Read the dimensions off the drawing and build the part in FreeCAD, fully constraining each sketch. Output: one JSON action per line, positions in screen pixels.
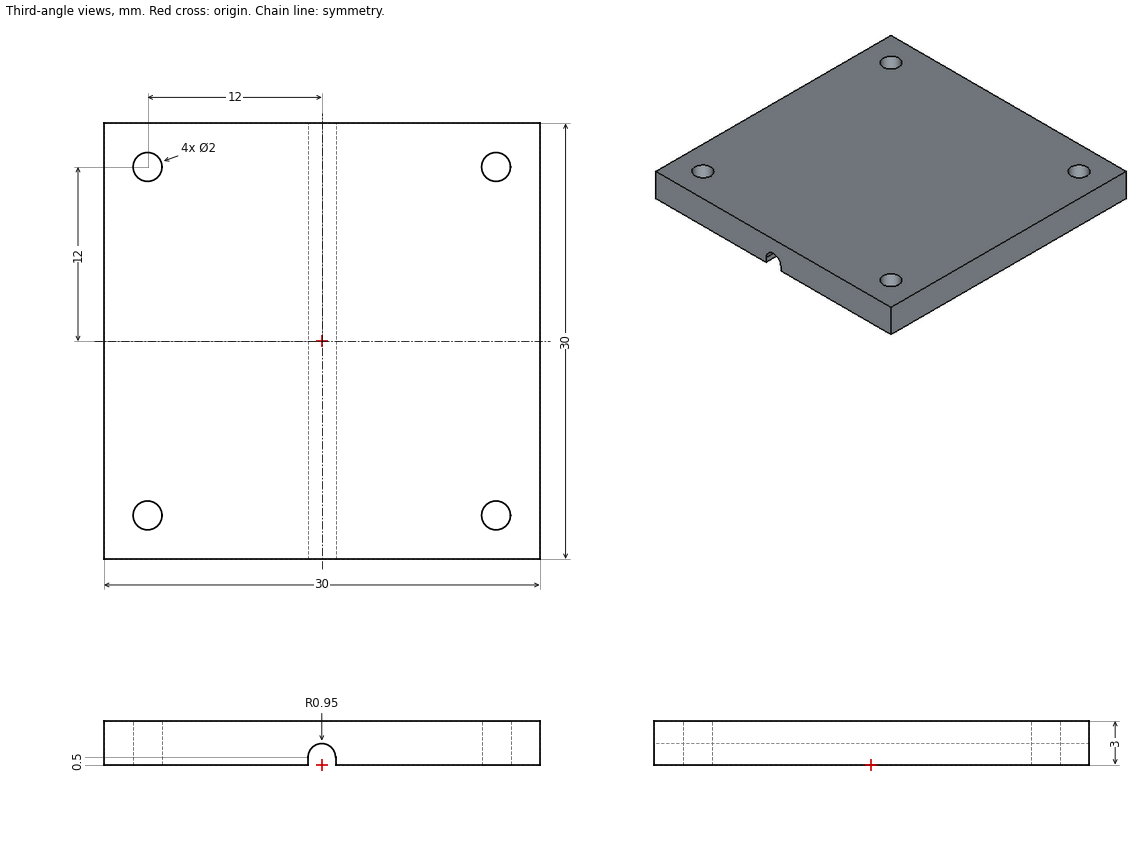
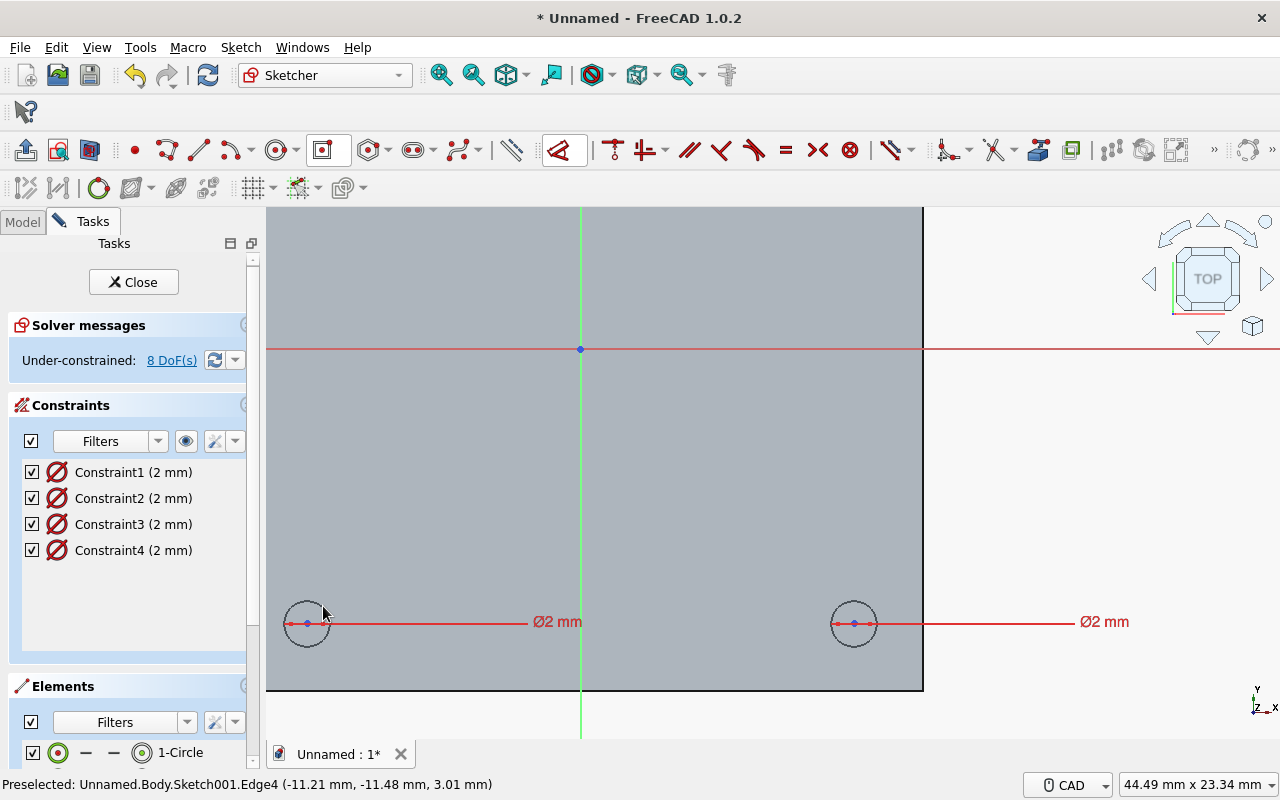
{"action": "scroll", "coordinate": [855, 624], "scroll_direction": "down", "scroll_amount": 3}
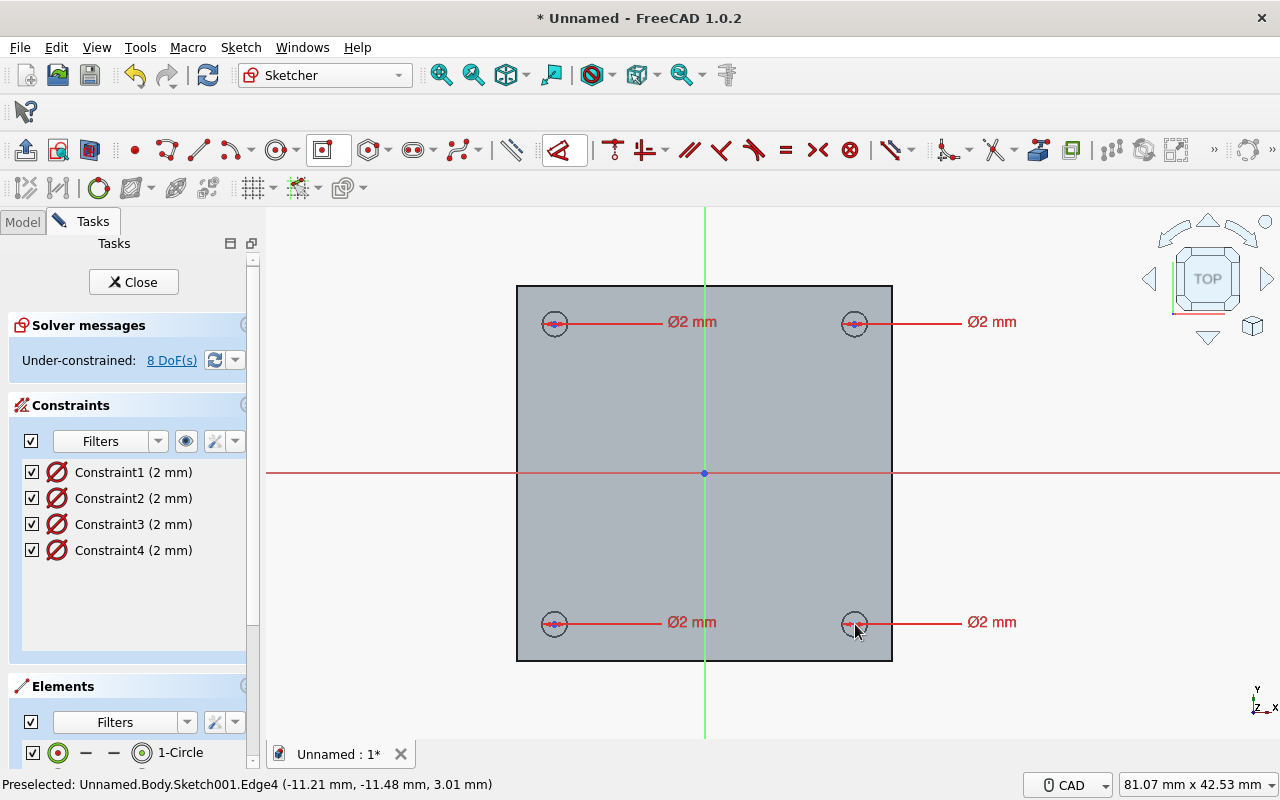
{"action": "left_click", "coordinate": [555, 324]}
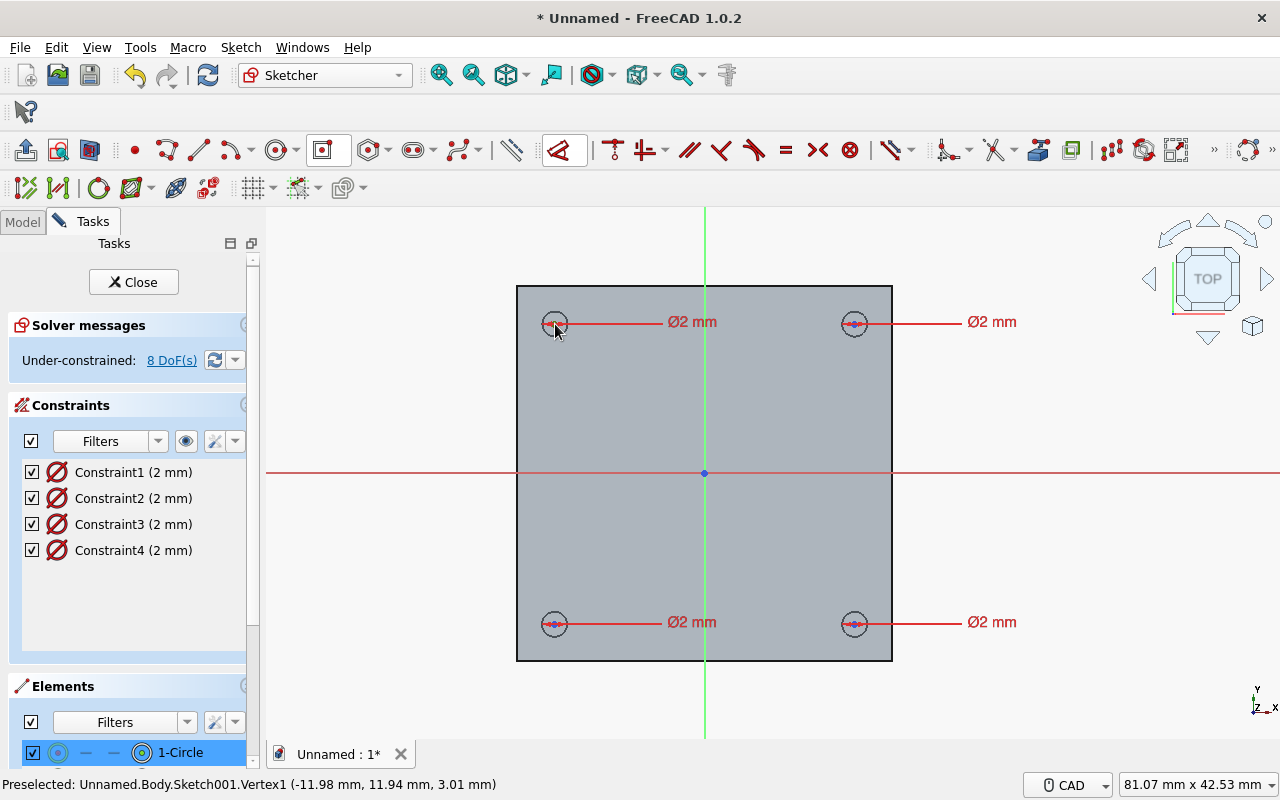
{"action": "left_click", "coordinate": [855, 324]}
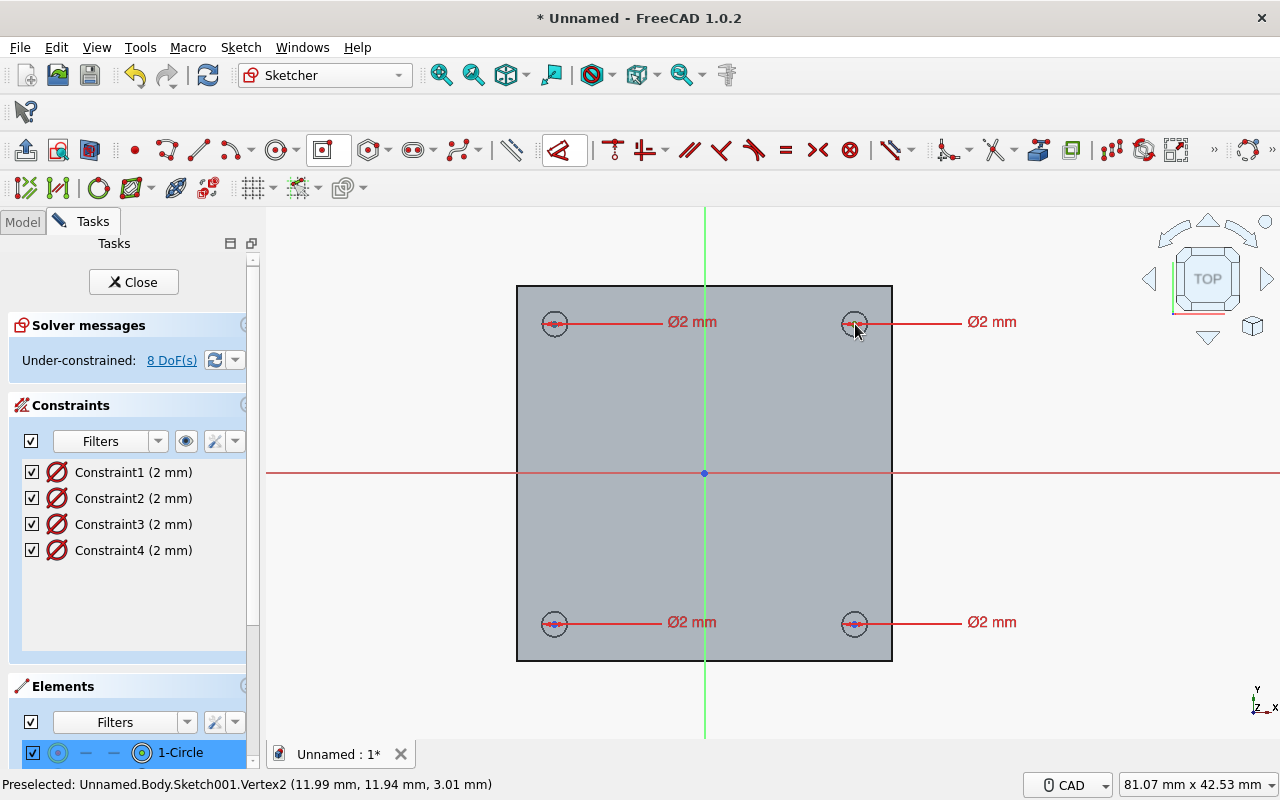
{"action": "left_click", "coordinate": [705, 677]}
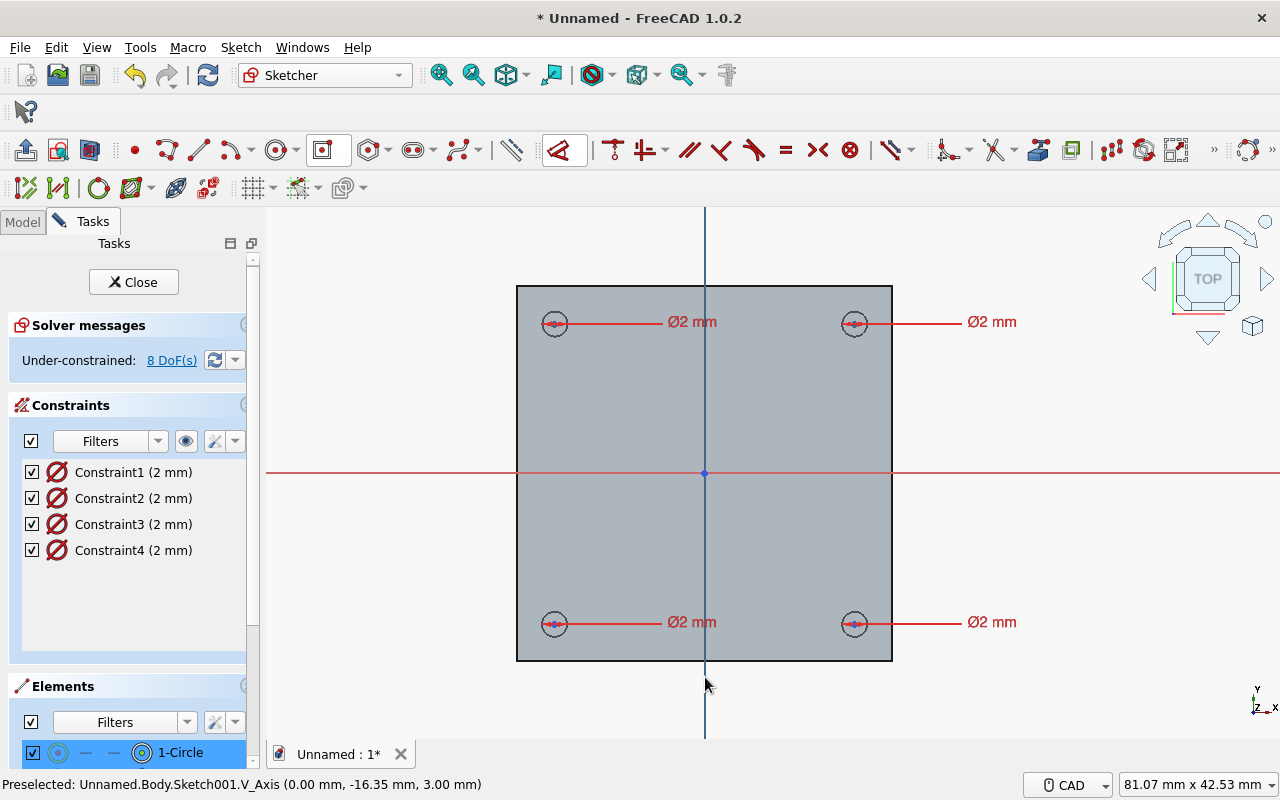
{"action": "left_click", "coordinate": [818, 150]}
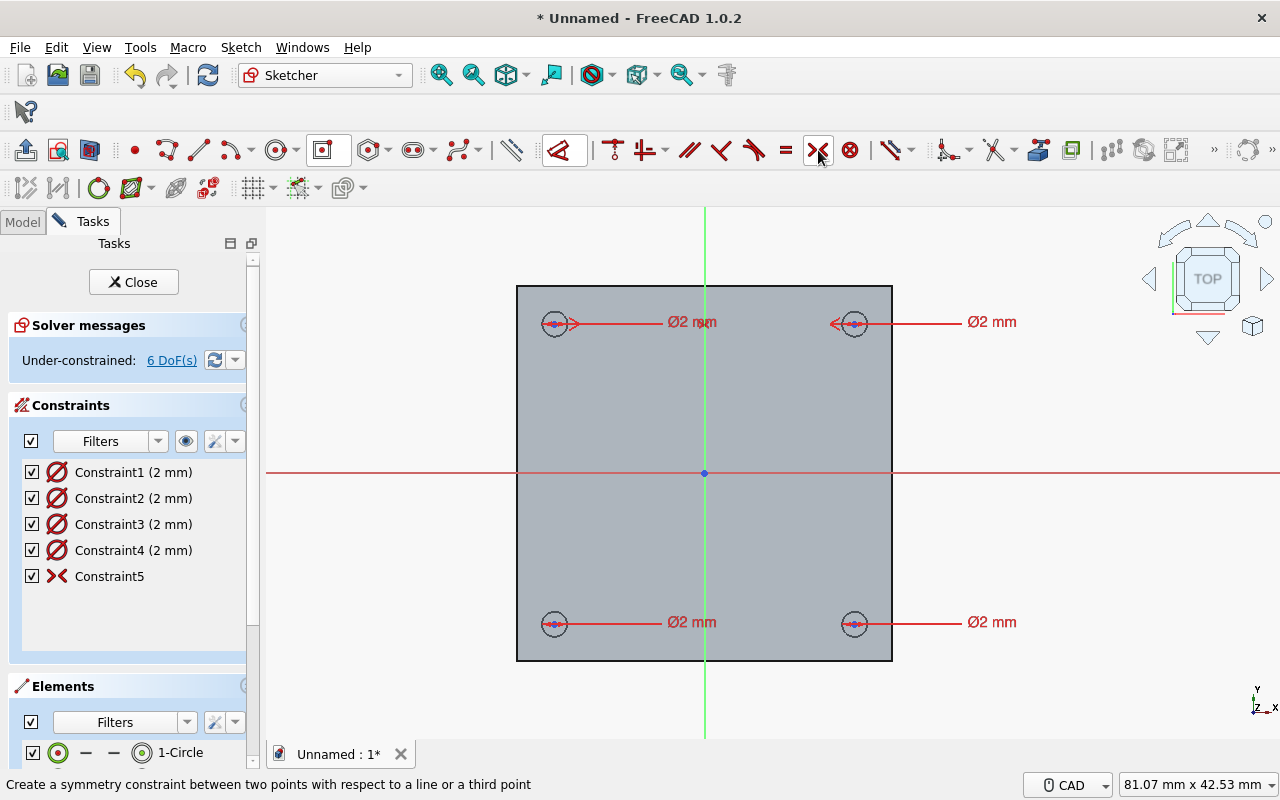
{"action": "left_click", "coordinate": [855, 324]}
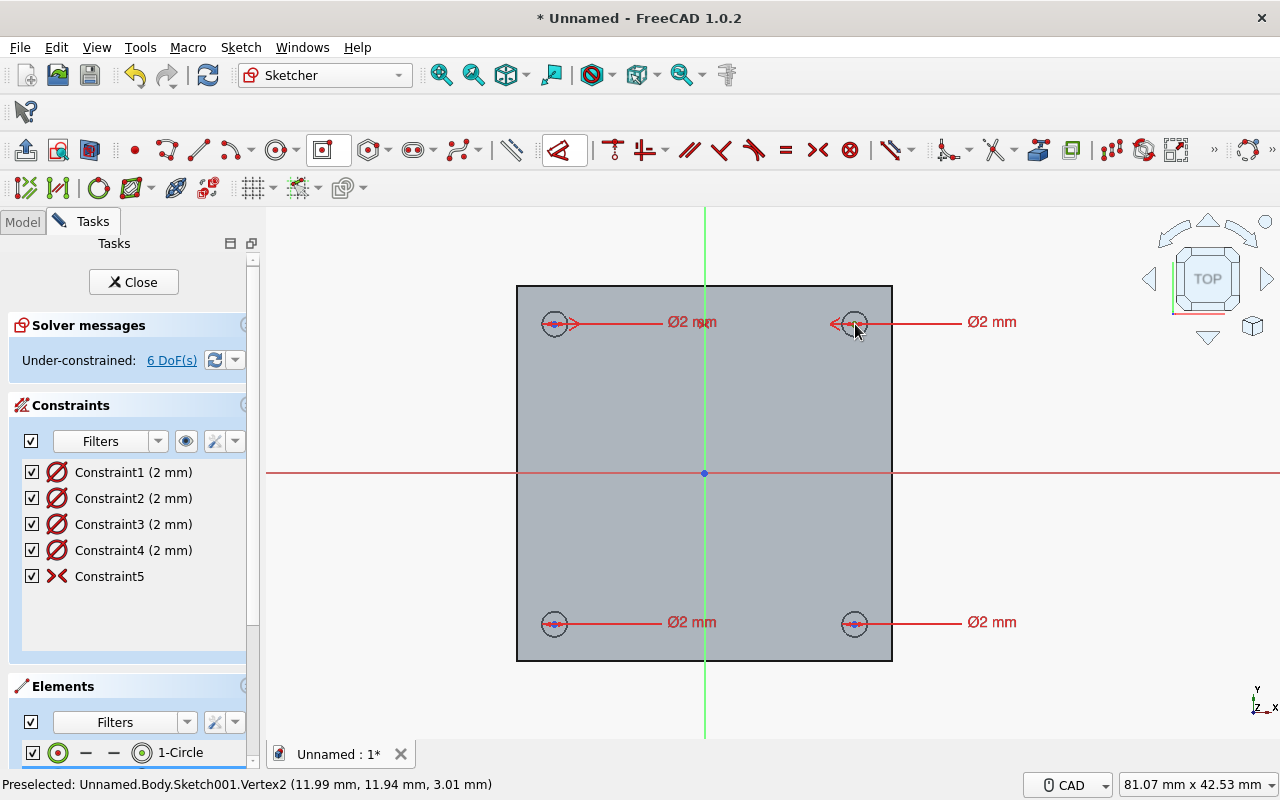
{"action": "left_click", "coordinate": [855, 624]}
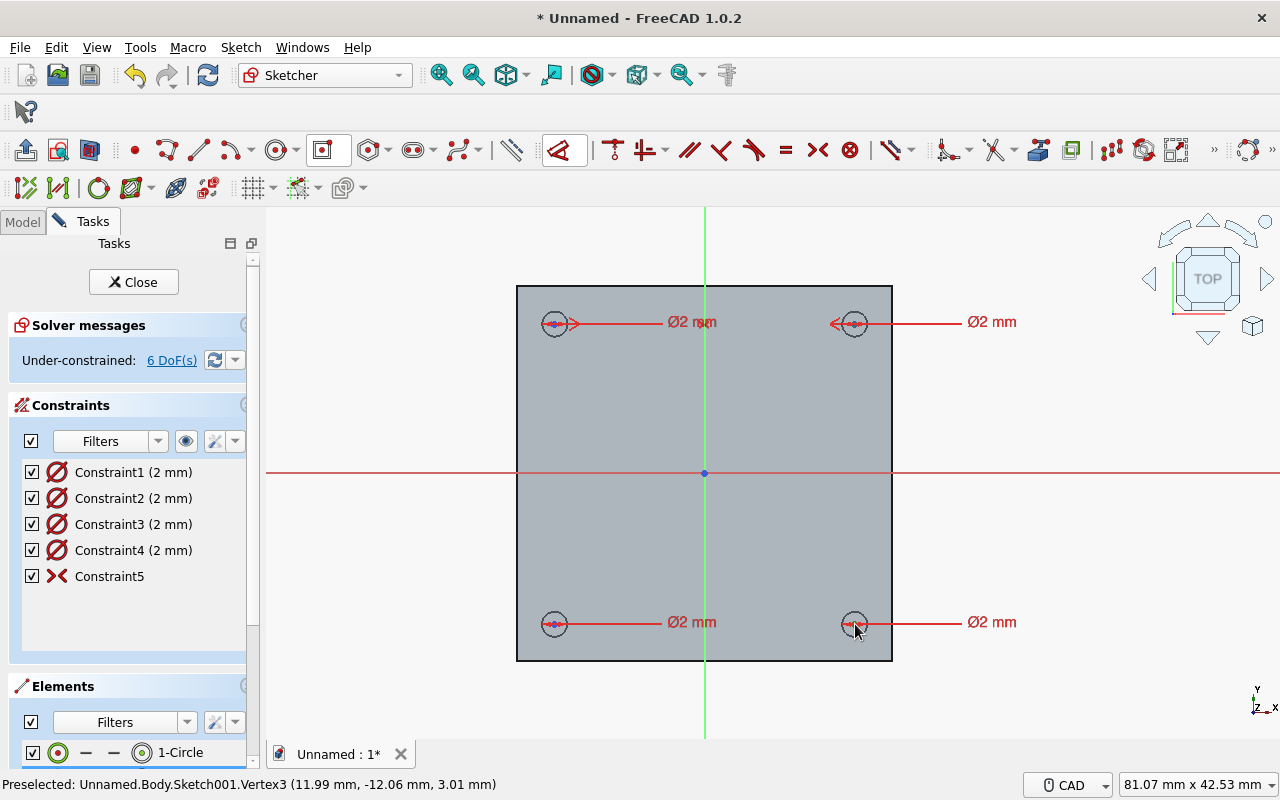
{"action": "left_click", "coordinate": [353, 473]}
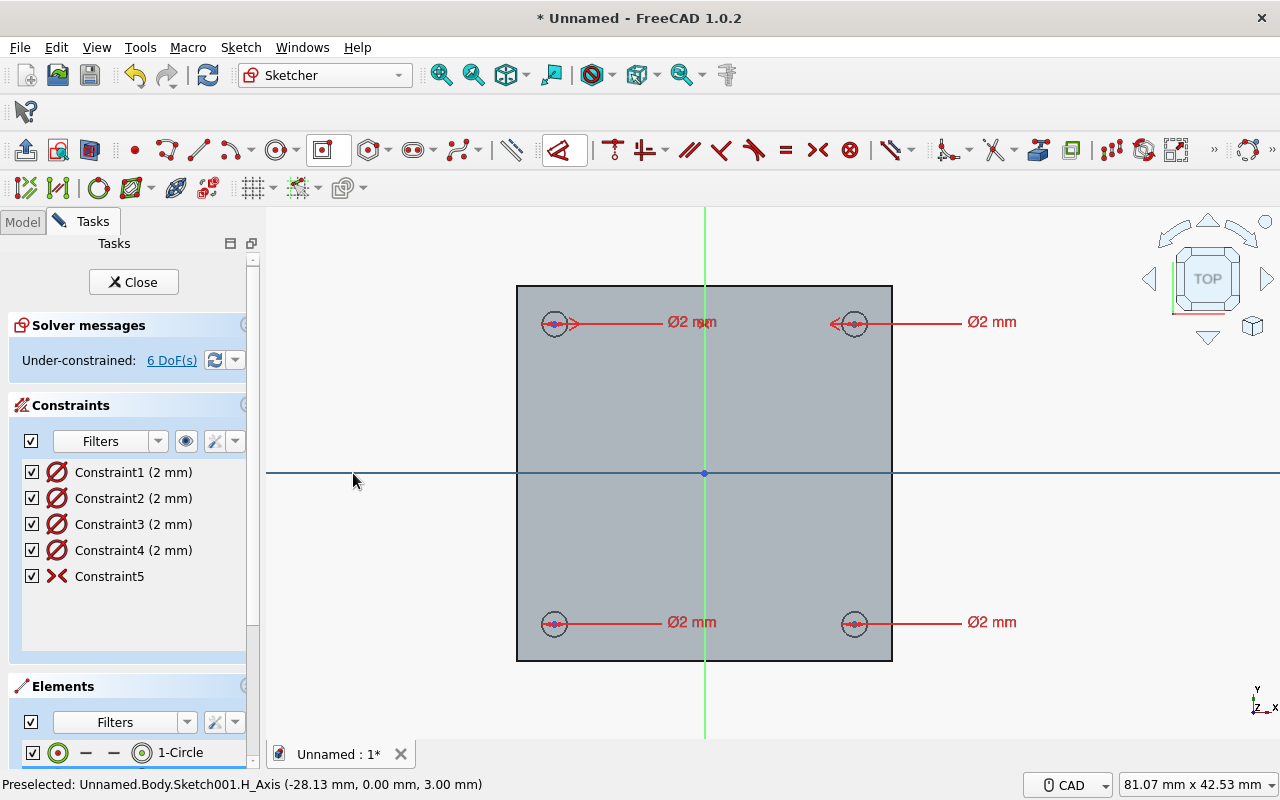
{"action": "left_click", "coordinate": [818, 150]}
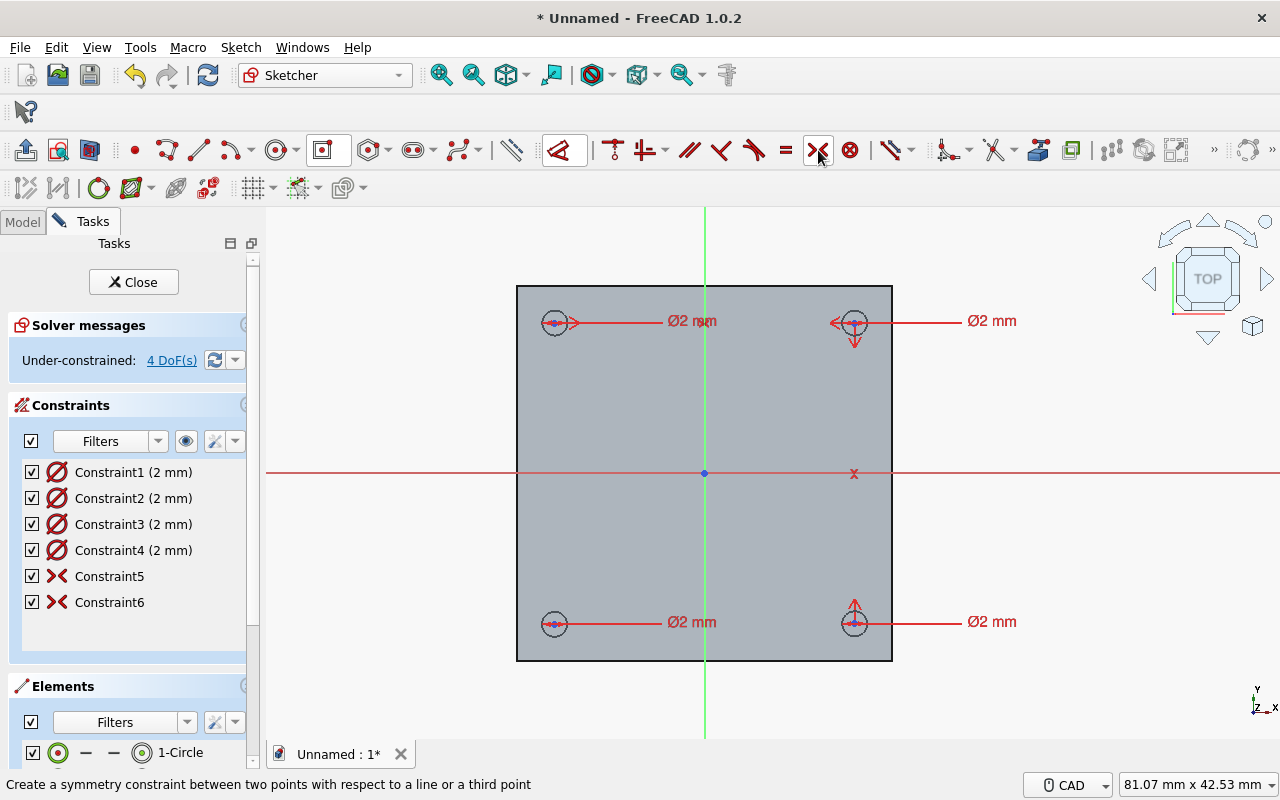
{"action": "left_click", "coordinate": [555, 323]}